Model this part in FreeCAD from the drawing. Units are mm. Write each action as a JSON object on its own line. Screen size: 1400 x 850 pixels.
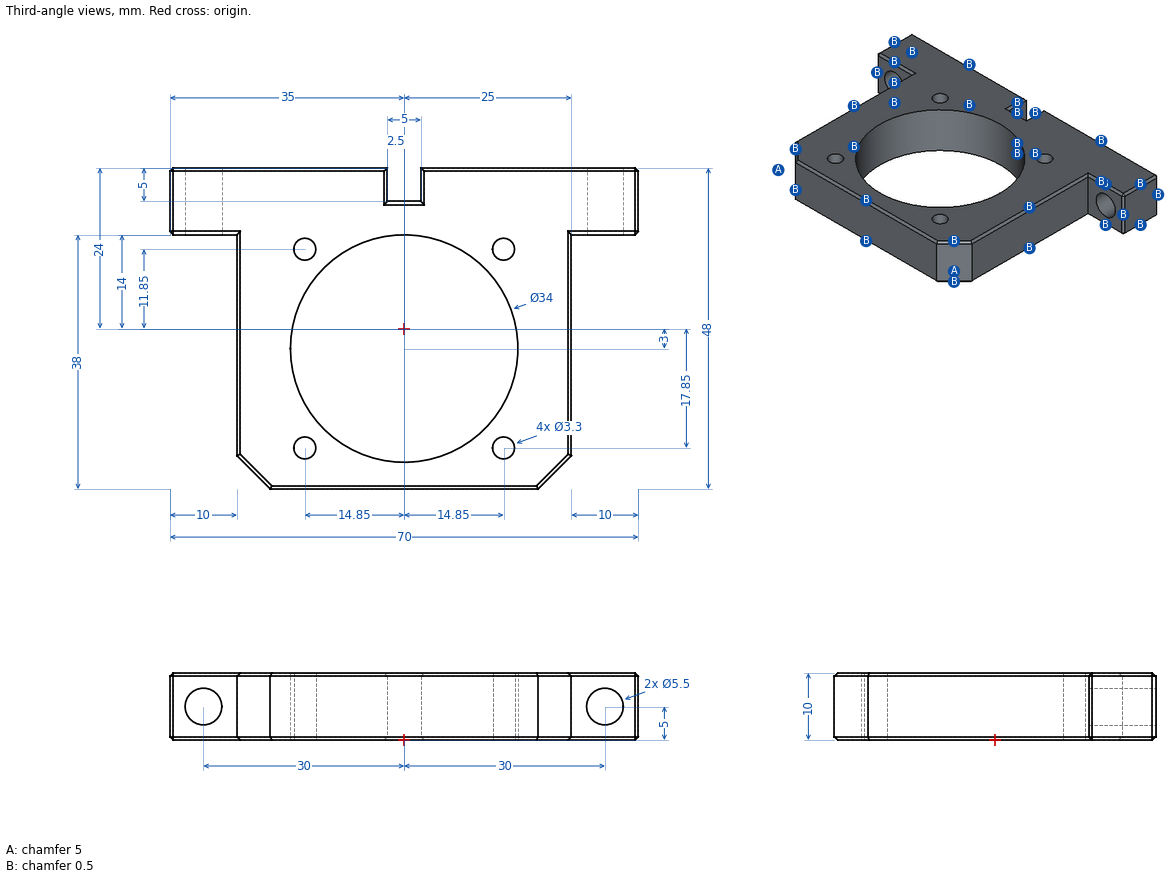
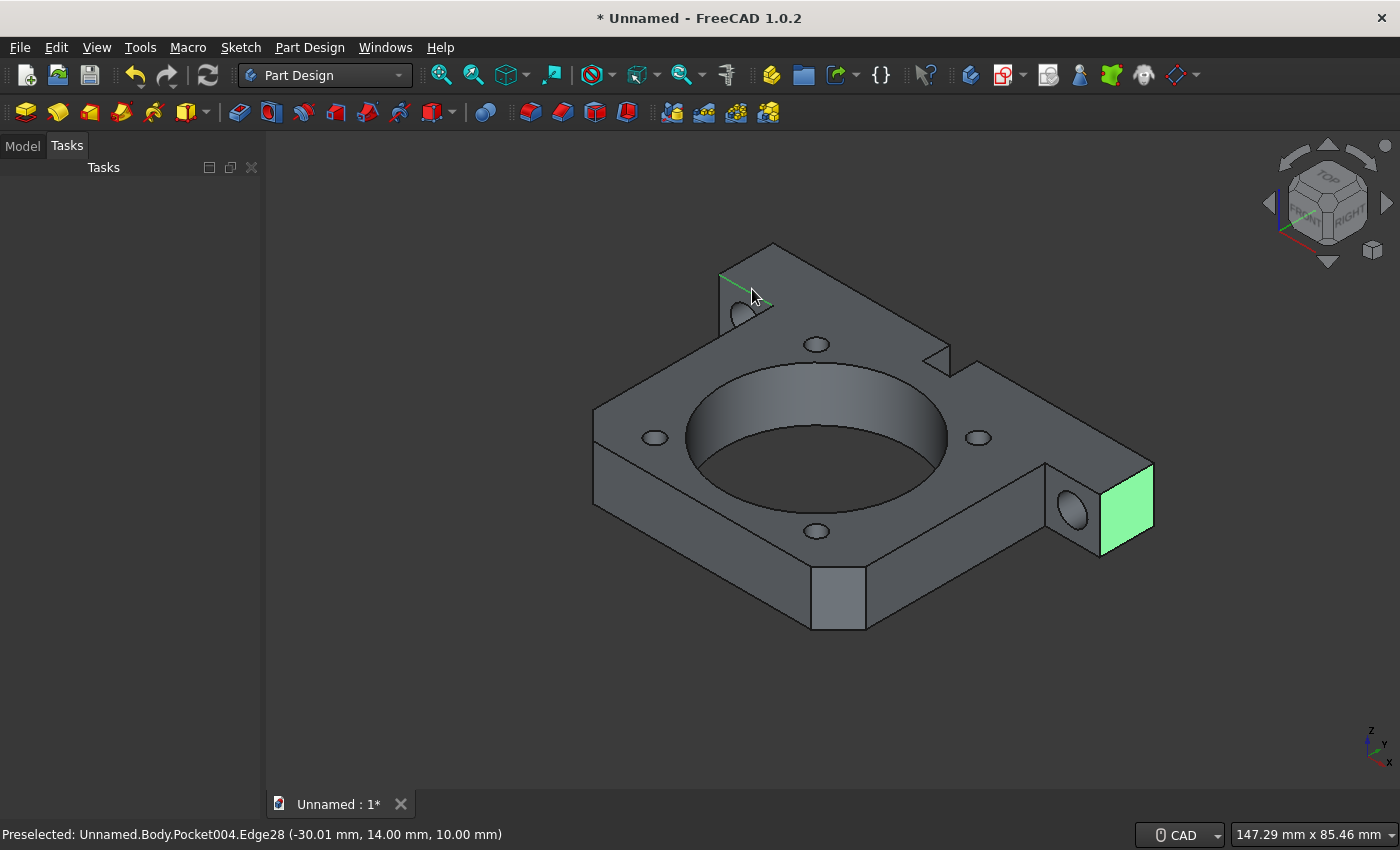
{"action": "left_click", "coordinate": [1073, 478], "text": "ctrl"}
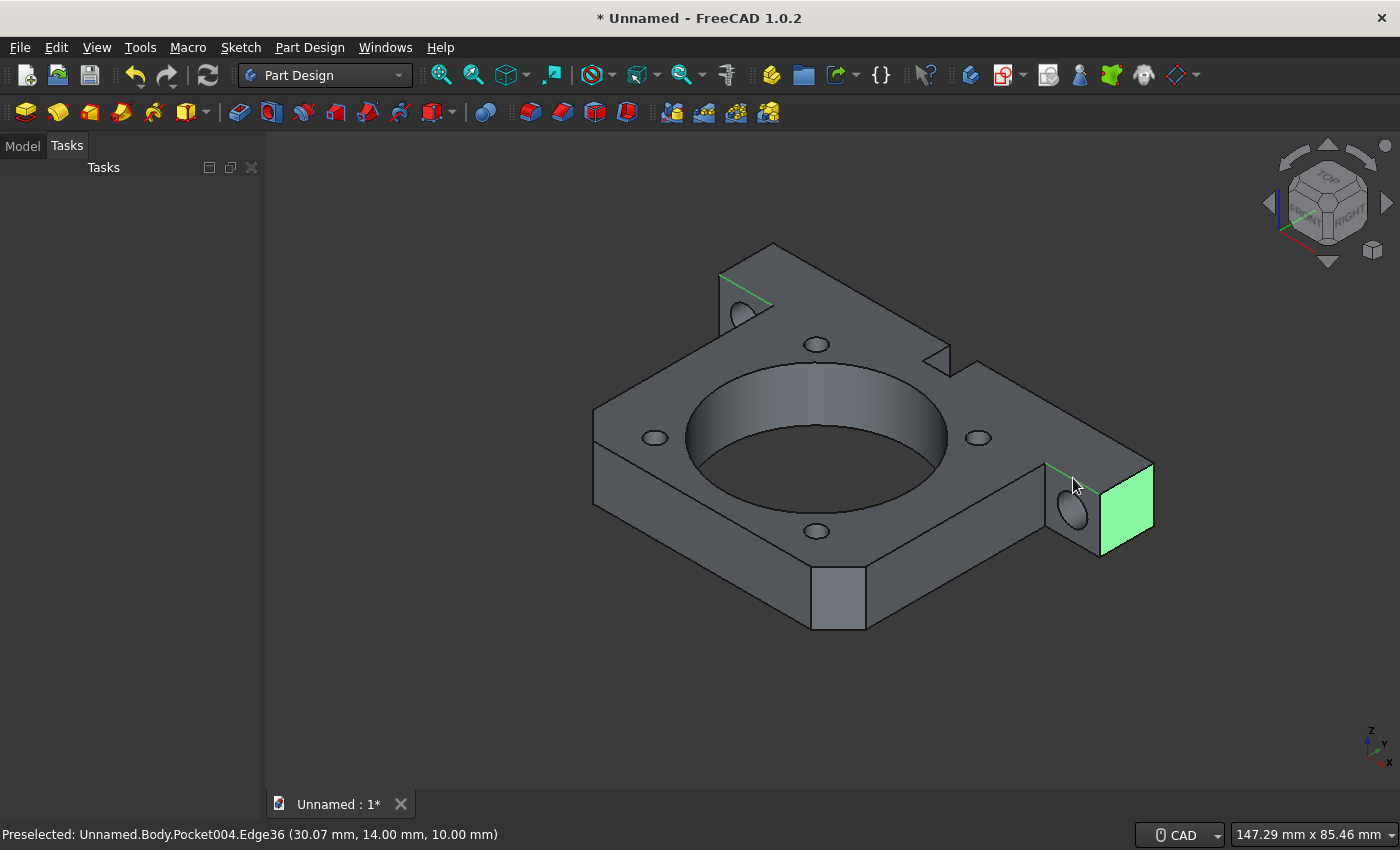
{"action": "left_click", "coordinate": [955, 514], "text": "ctrl"}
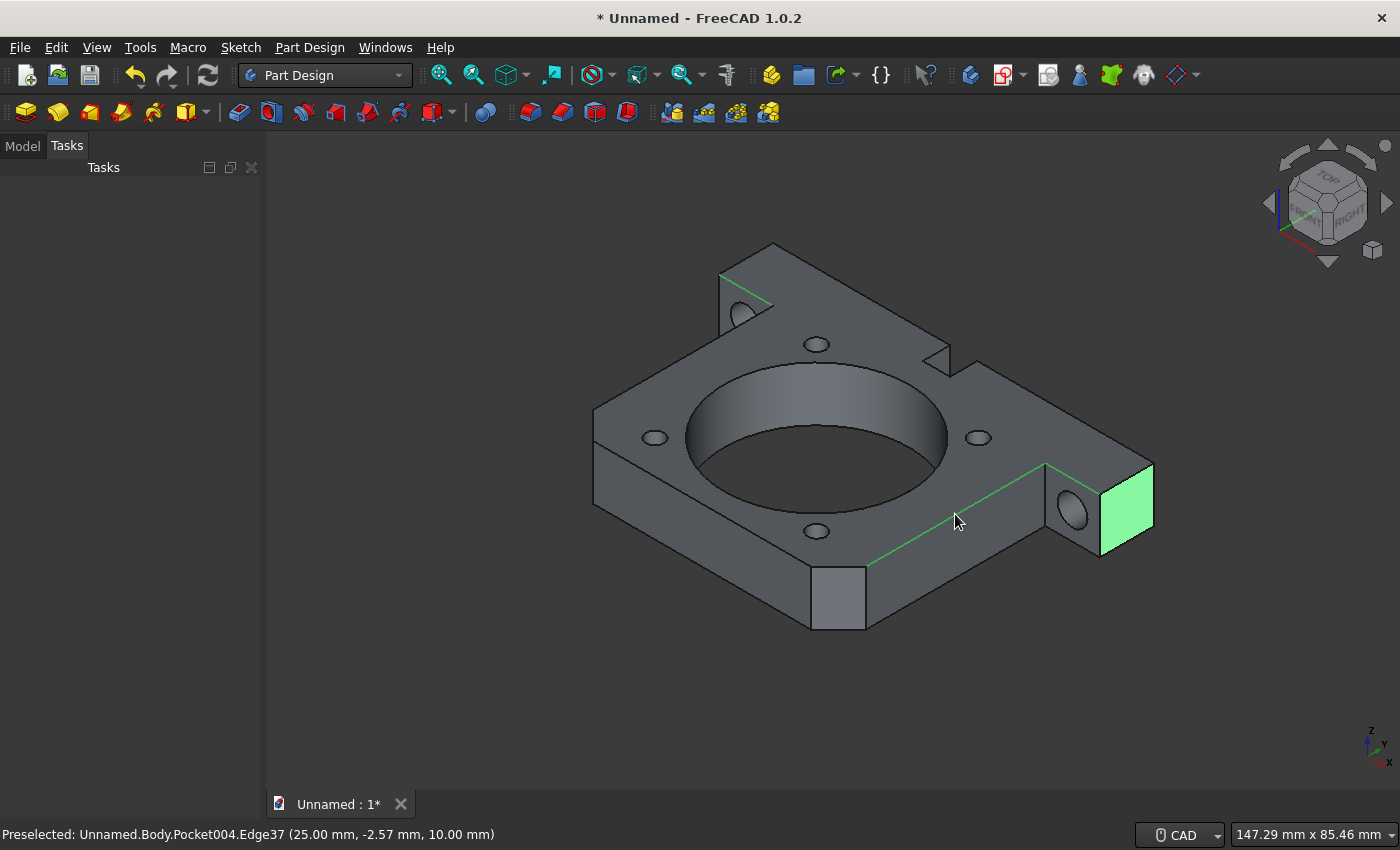
{"action": "left_click", "coordinate": [702, 503], "text": "ctrl"}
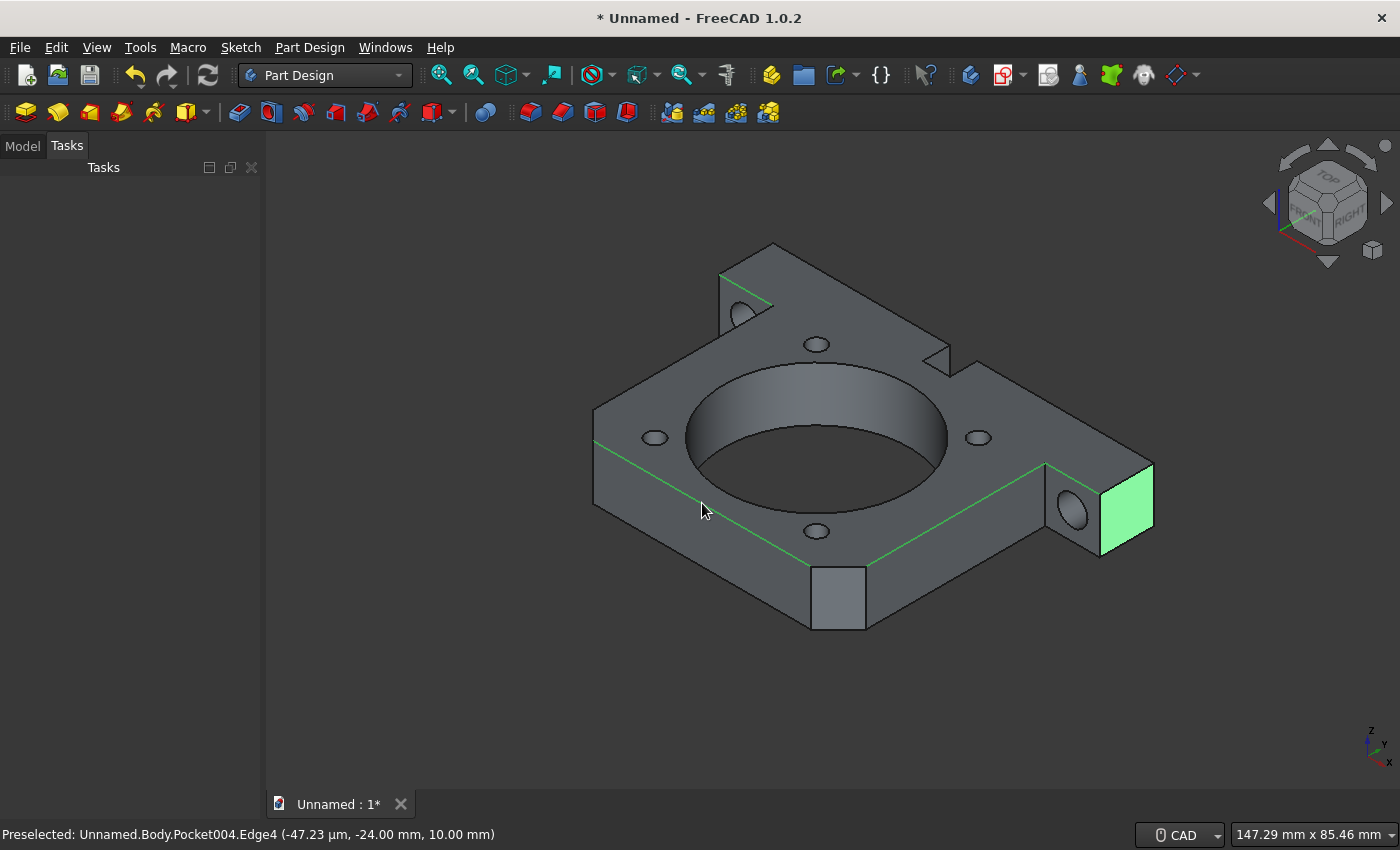
{"action": "left_click", "coordinate": [838, 566], "text": "ctrl"}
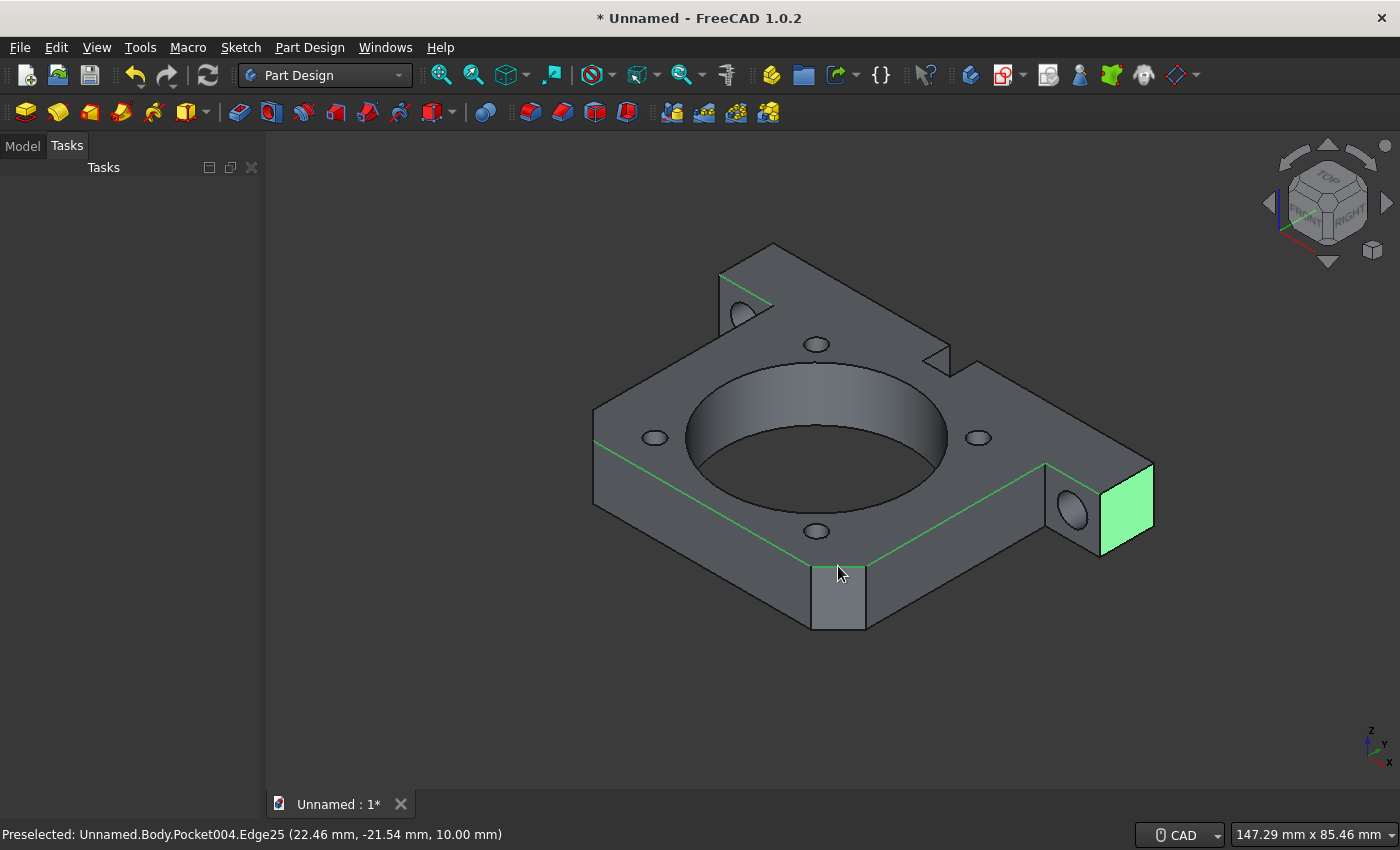
{"action": "left_click", "coordinate": [936, 352], "text": "ctrl"}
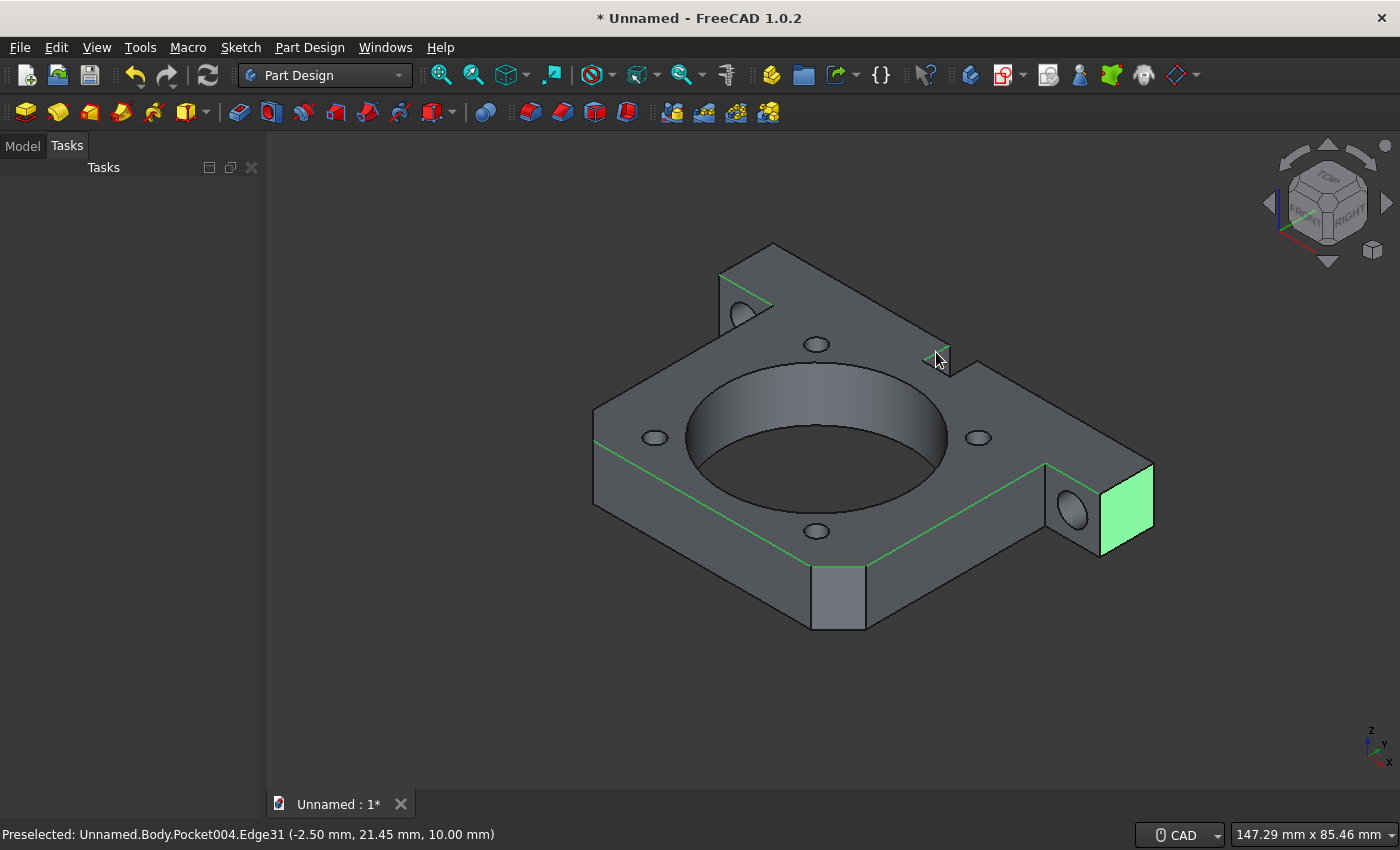
{"action": "key", "text": "2"}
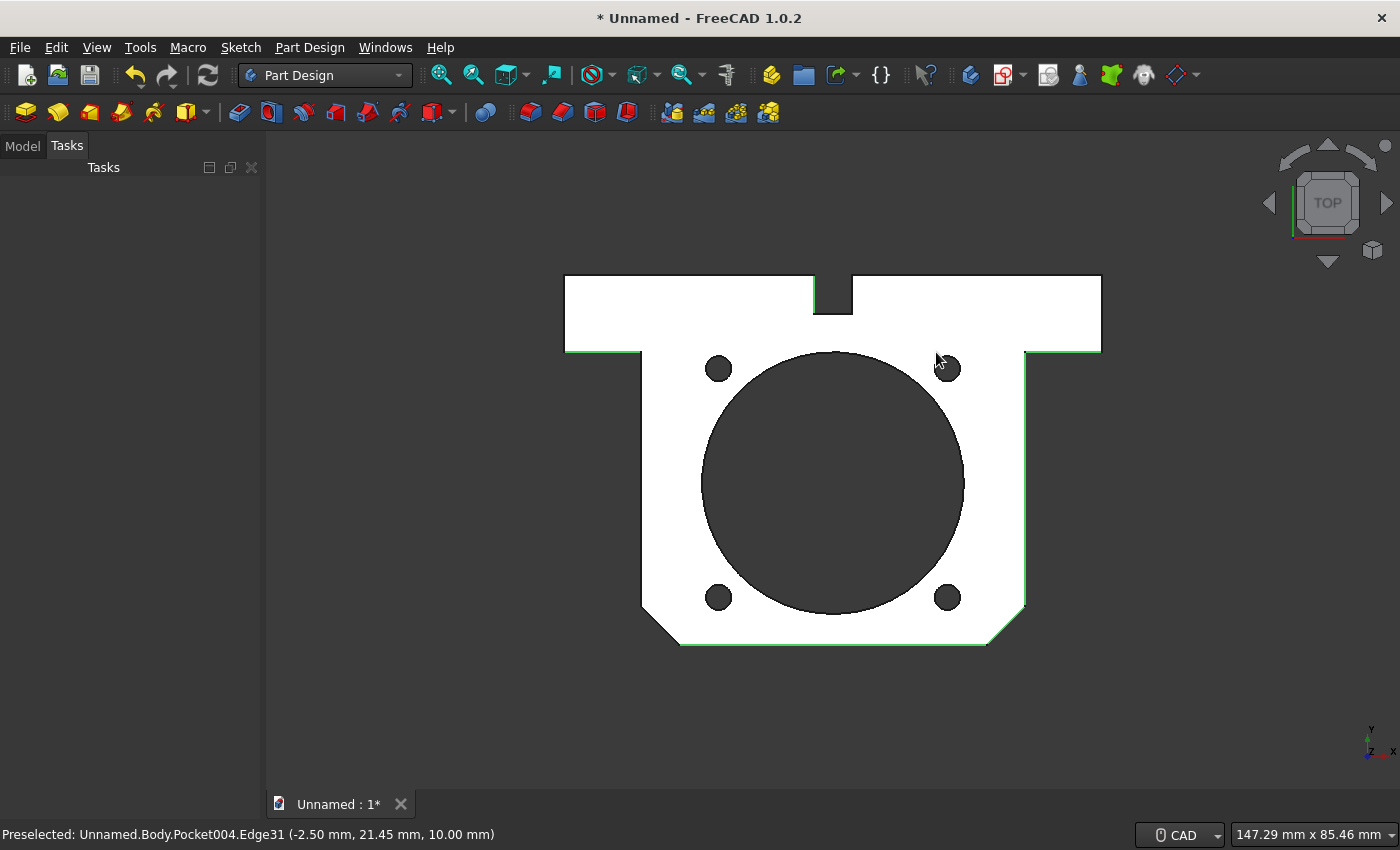
{"action": "left_click", "coordinate": [977, 274], "text": "ctrl"}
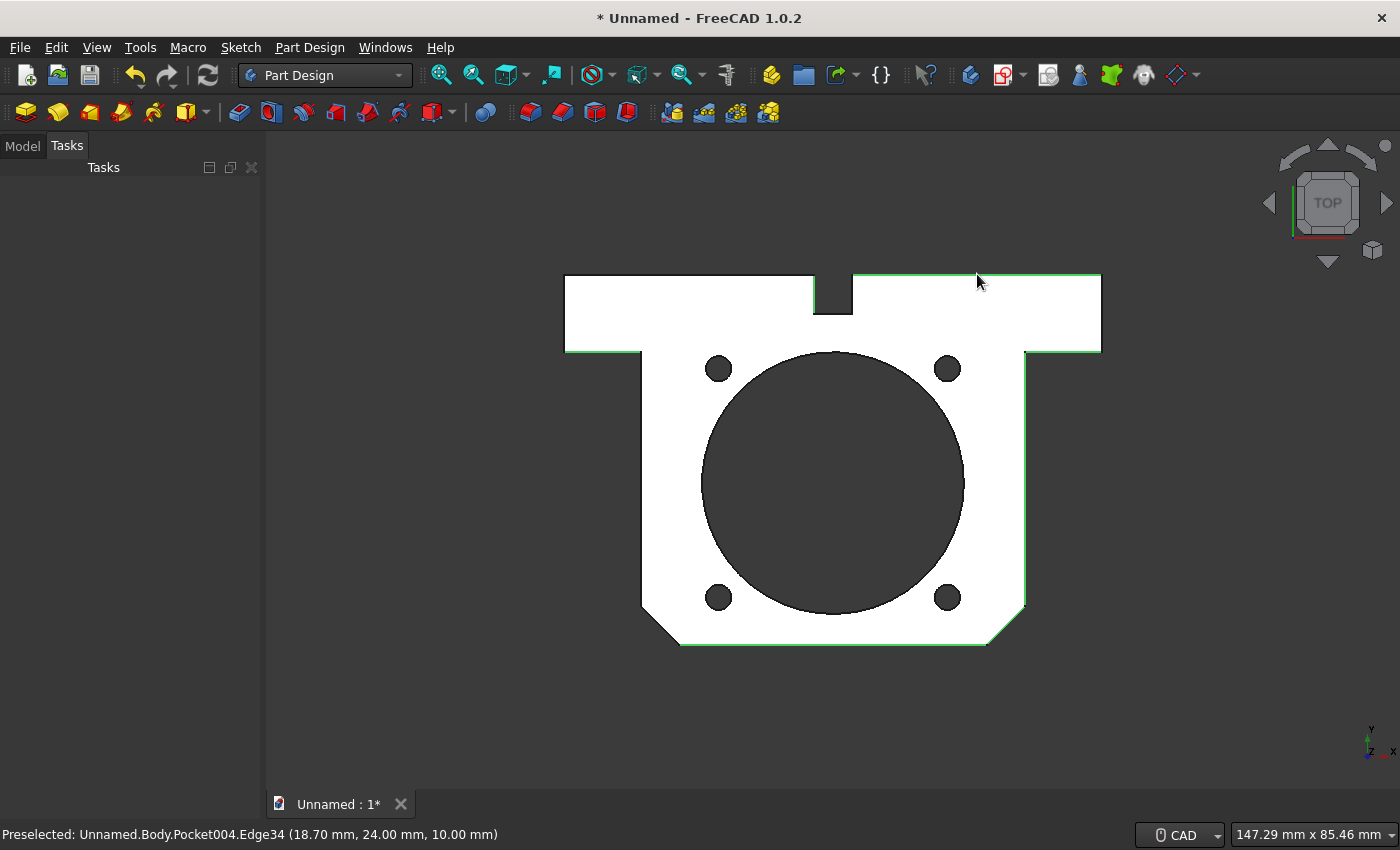
{"action": "left_click", "coordinate": [641, 478], "text": "ctrl"}